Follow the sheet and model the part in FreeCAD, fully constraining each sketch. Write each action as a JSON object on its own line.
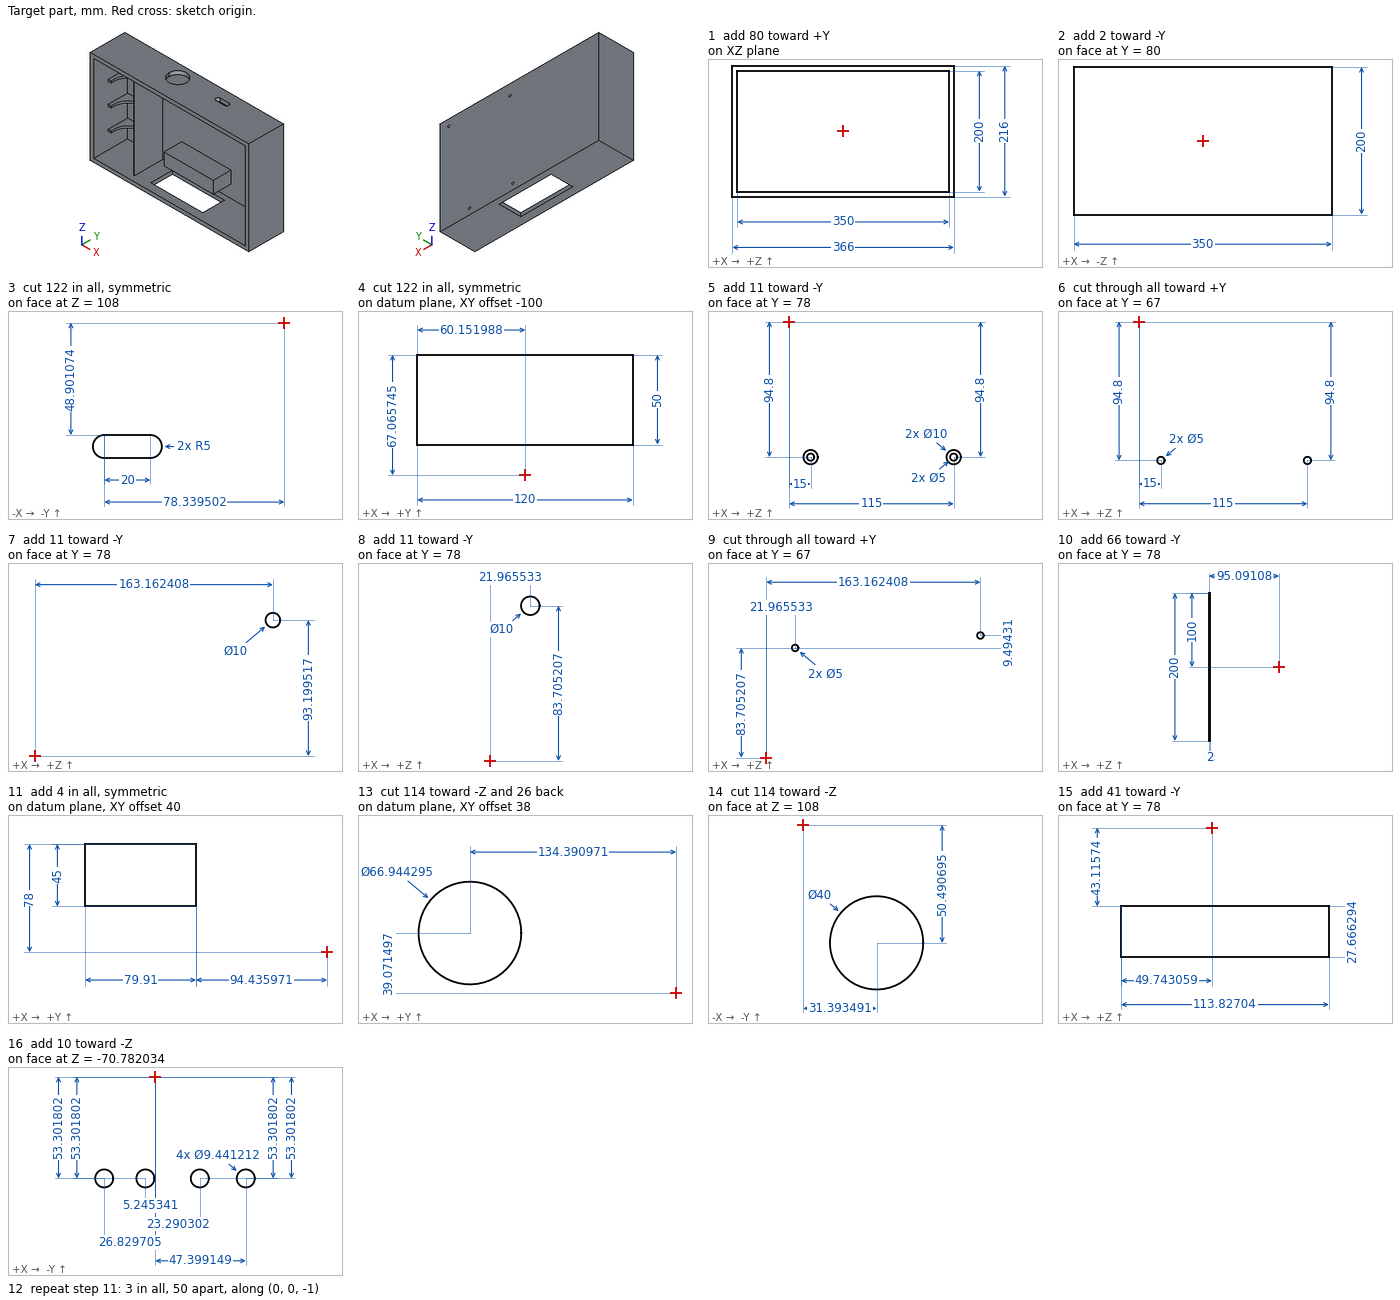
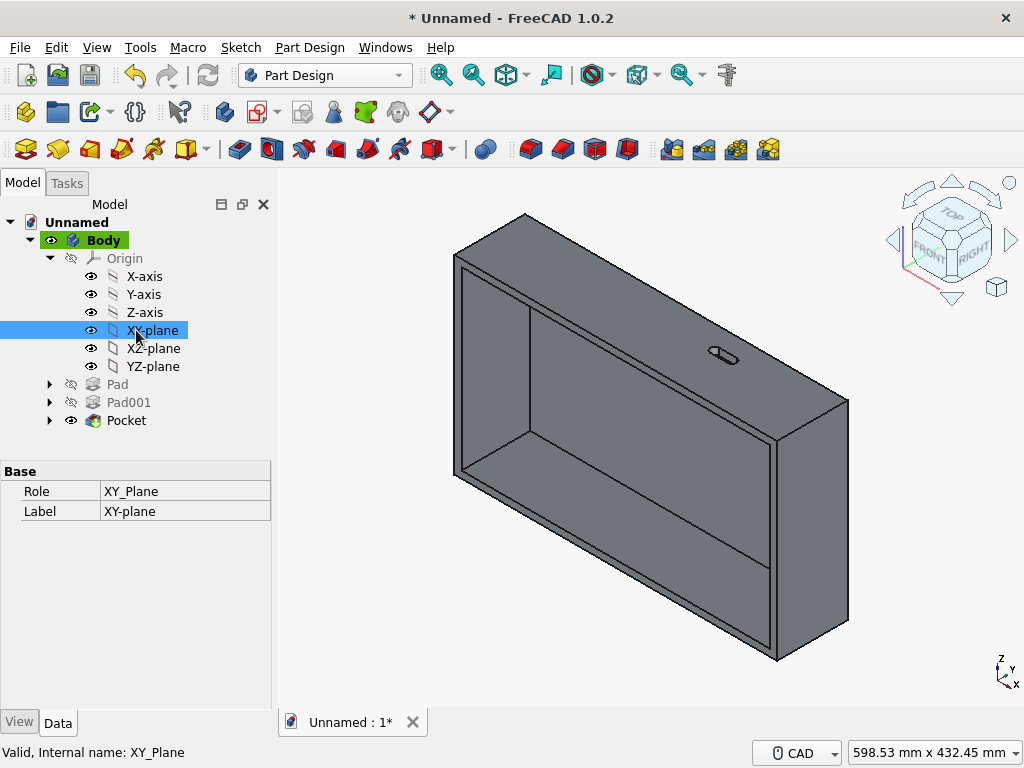
{"action": "left_click", "coordinate": [430, 112]}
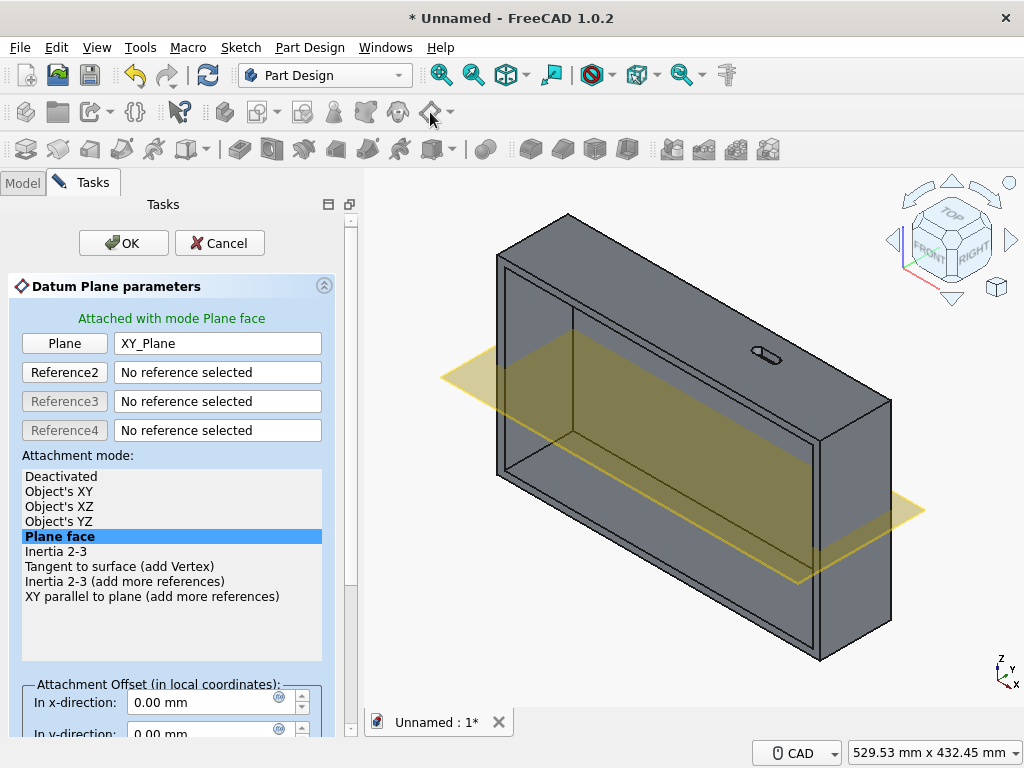
{"action": "scroll", "coordinate": [351, 475], "scroll_direction": "down", "scroll_amount": 2}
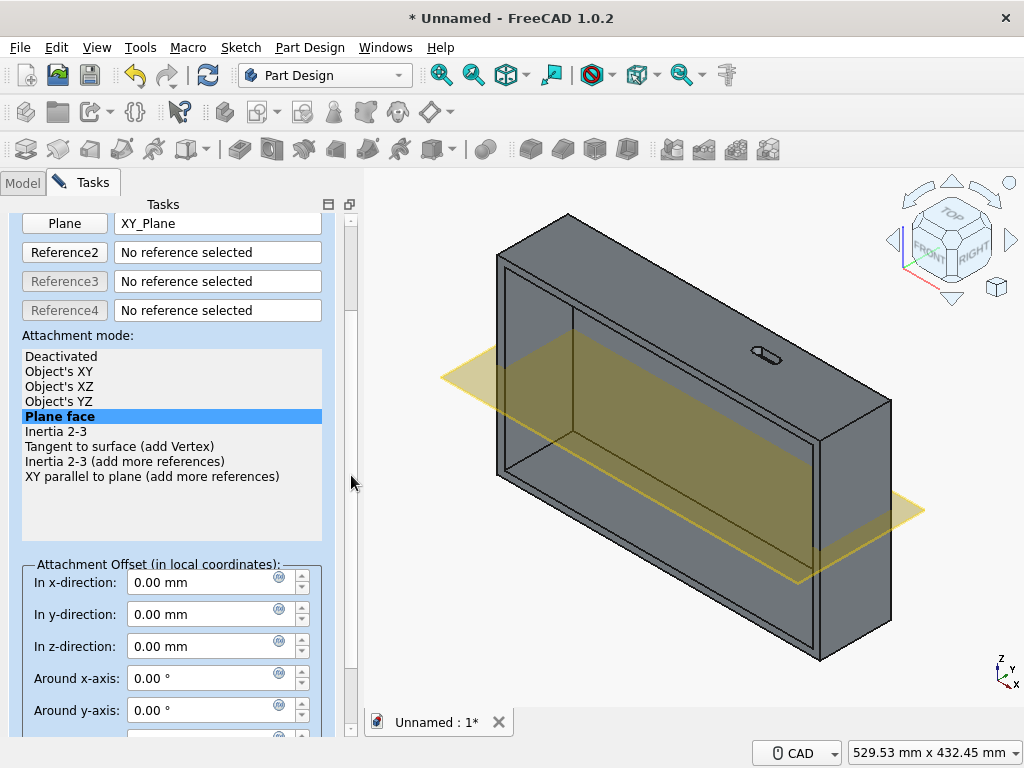
{"action": "triple_click", "coordinate": [210, 646]}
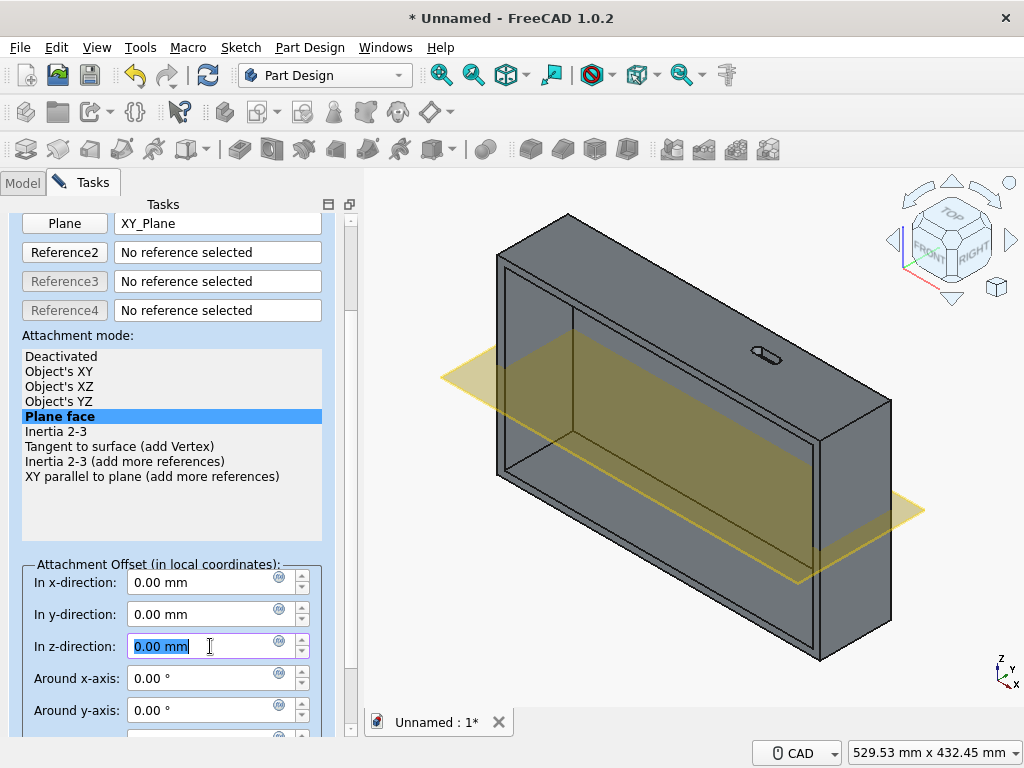
{"action": "type", "text": "-100"}
{"action": "key", "text": "Tab"}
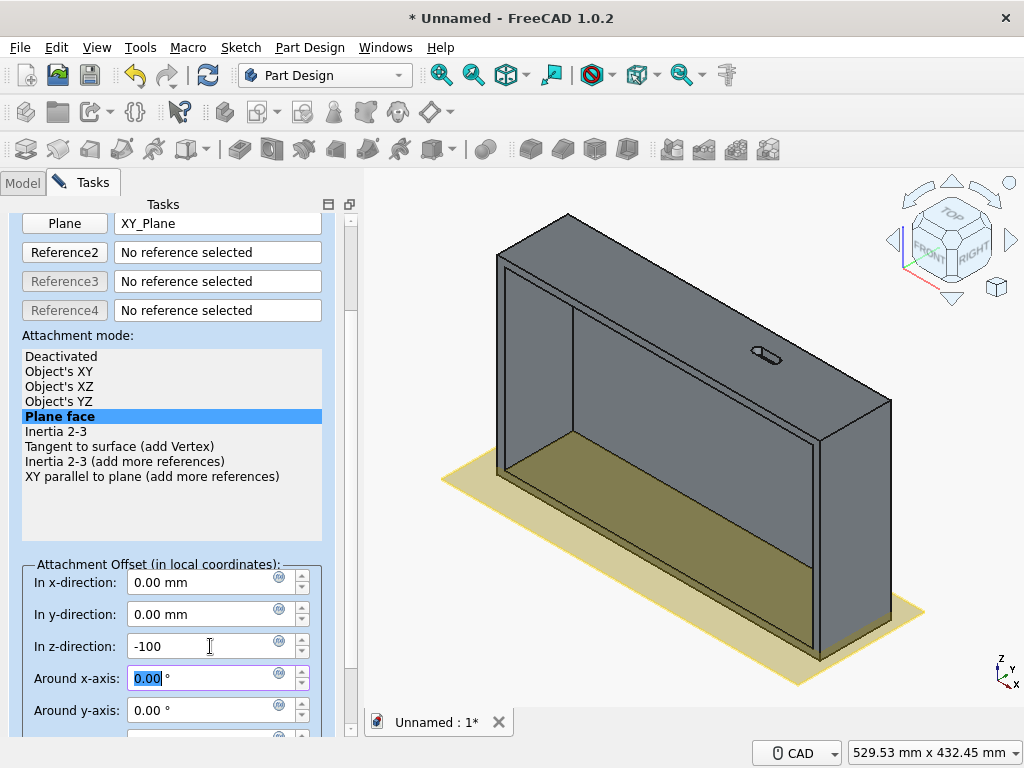
{"action": "scroll", "coordinate": [351, 475], "scroll_direction": "up", "scroll_amount": 3}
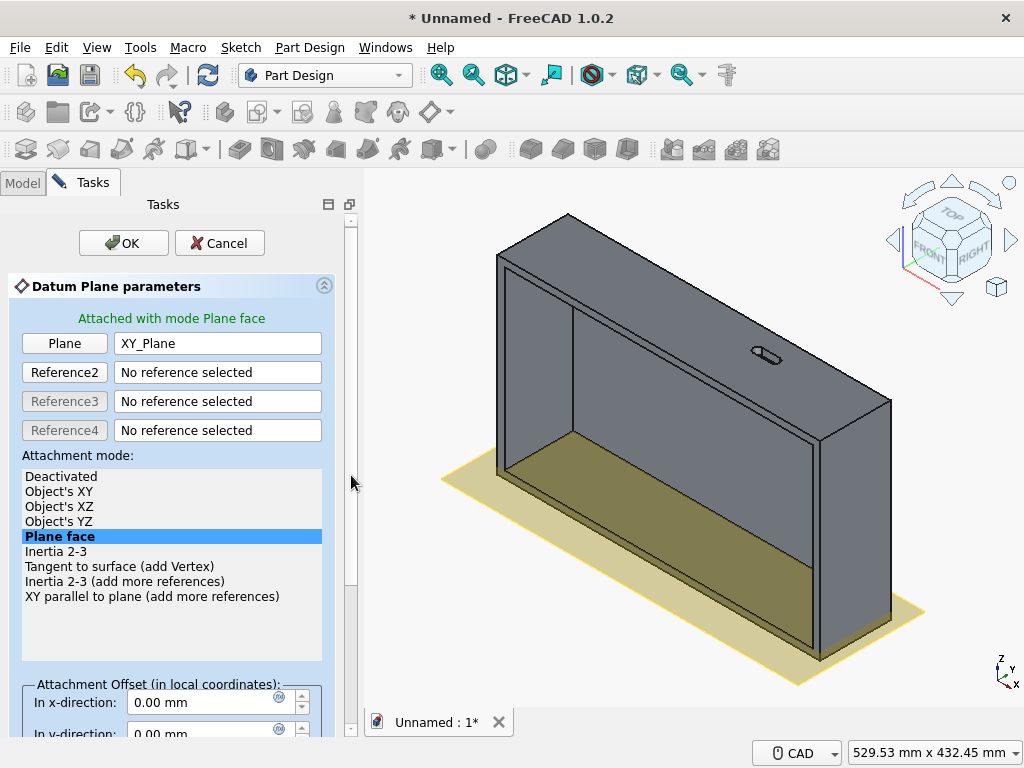
{"action": "left_click", "coordinate": [124, 243]}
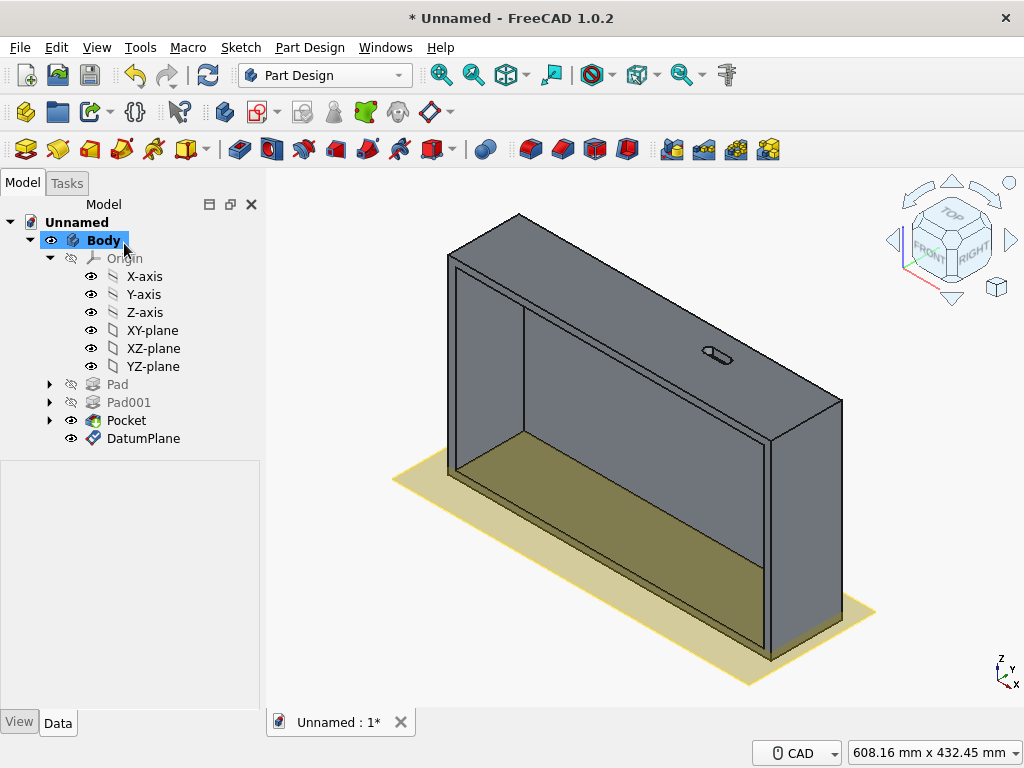
{"action": "left_click", "coordinate": [116, 438]}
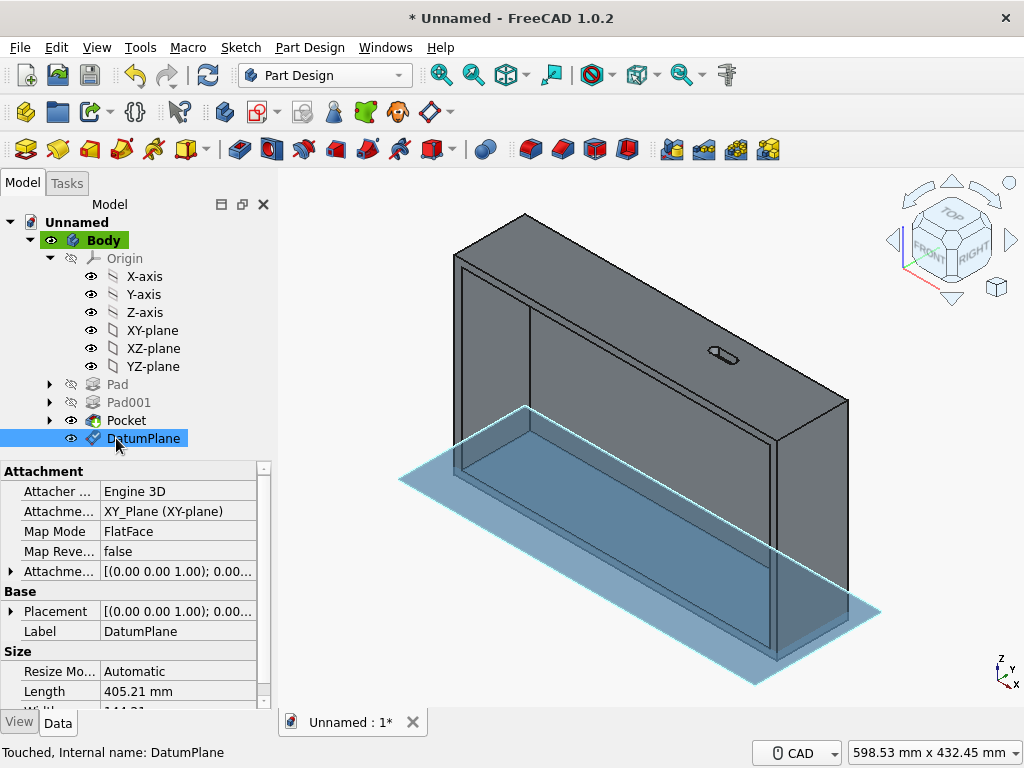
{"action": "left_click", "coordinate": [258, 112]}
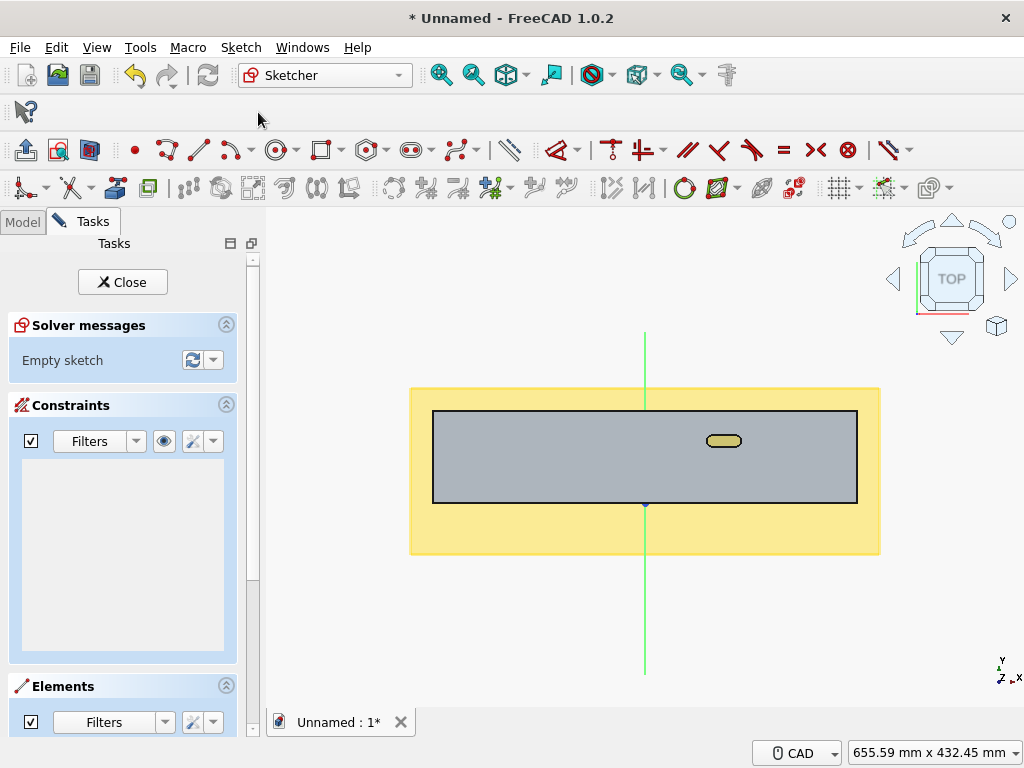
{"action": "key", "text": "q s"}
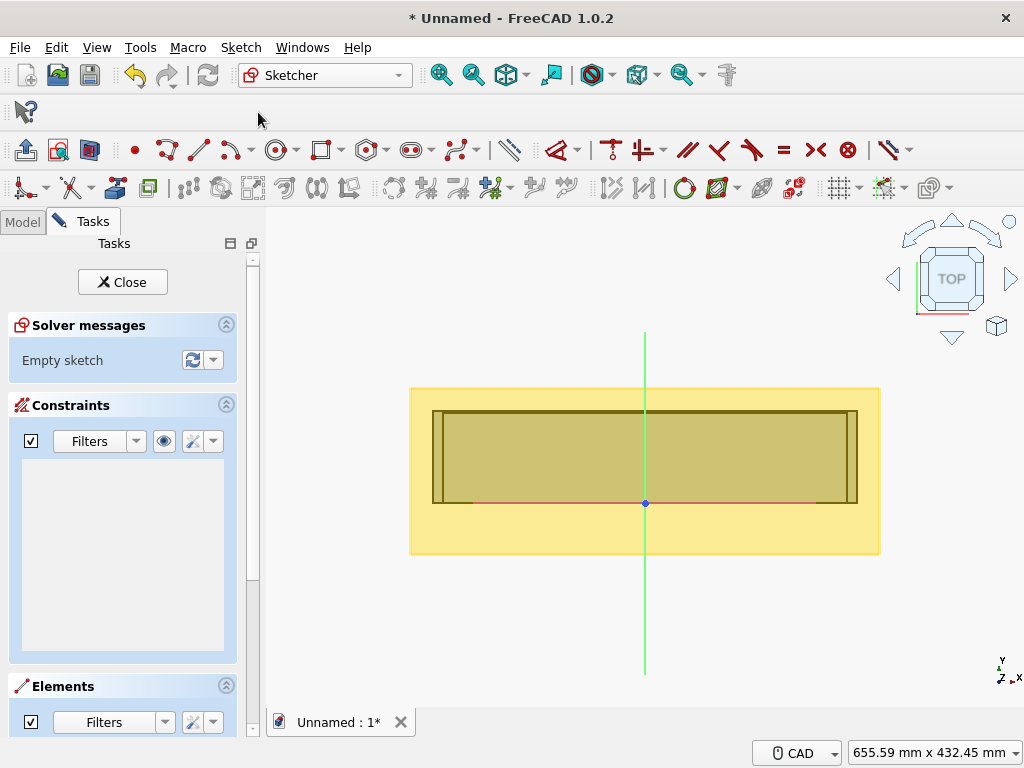
{"action": "scroll", "coordinate": [685, 469], "scroll_direction": "up", "scroll_amount": 5}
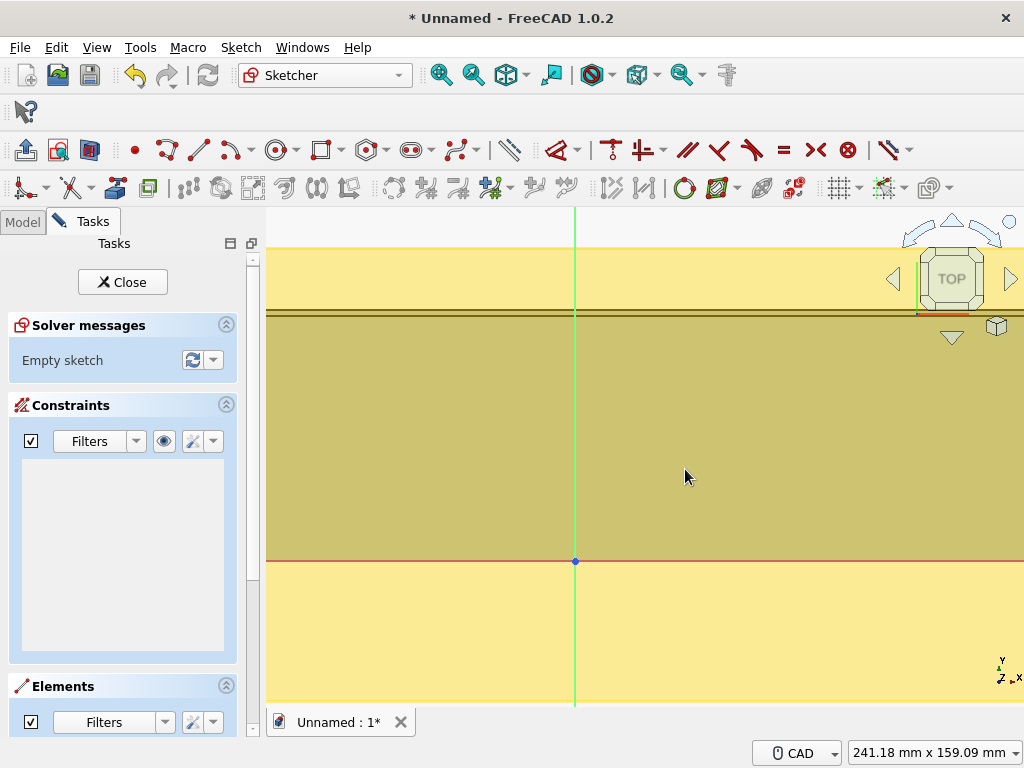
{"action": "left_click", "coordinate": [322, 150]}